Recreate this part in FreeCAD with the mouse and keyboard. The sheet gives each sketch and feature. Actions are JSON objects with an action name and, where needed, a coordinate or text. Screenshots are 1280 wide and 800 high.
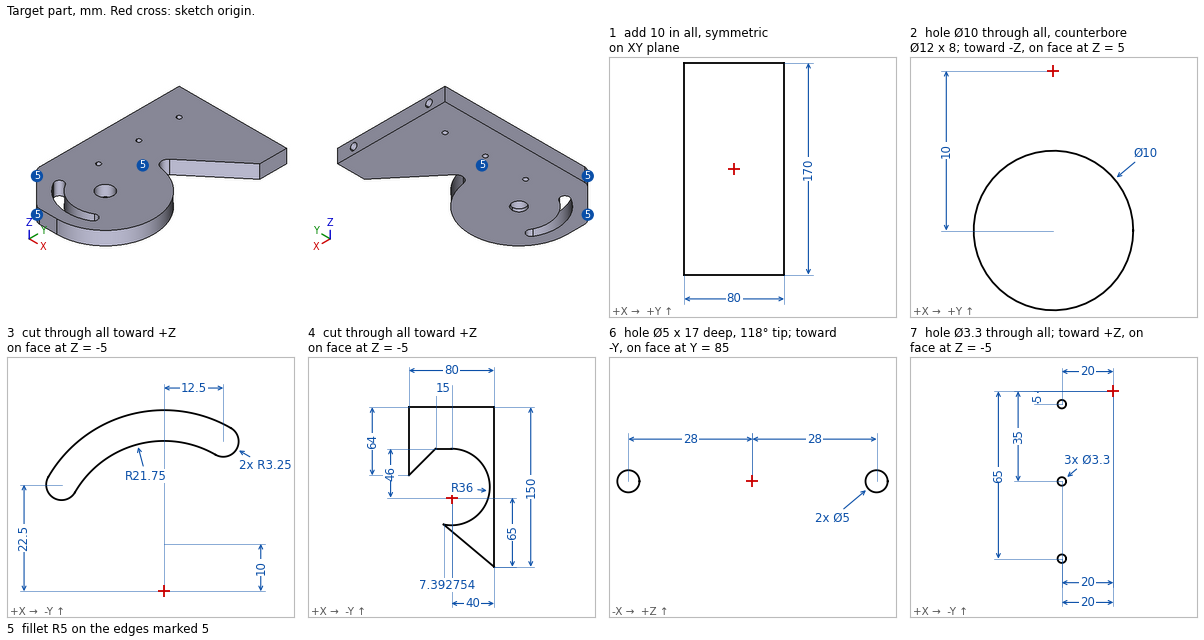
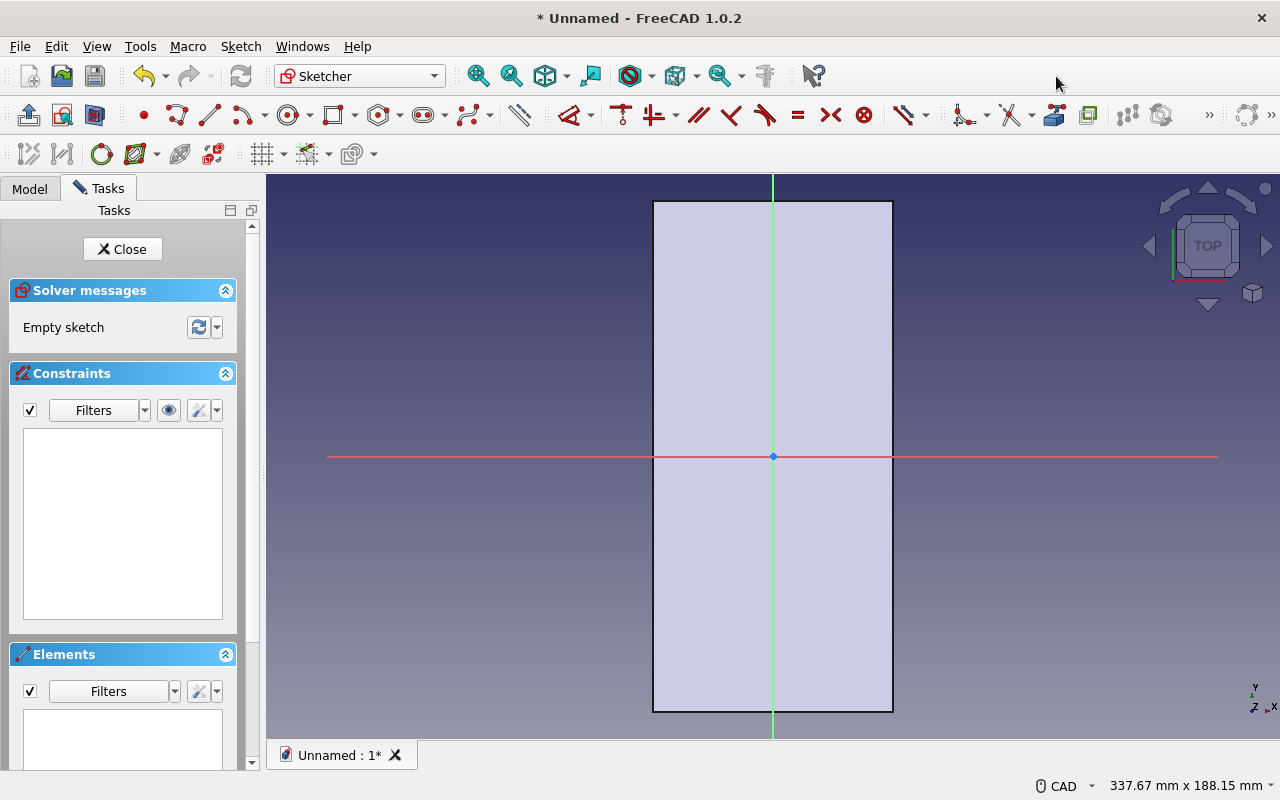
{"action": "scroll", "coordinate": [784, 483], "scroll_direction": "up", "scroll_amount": 10}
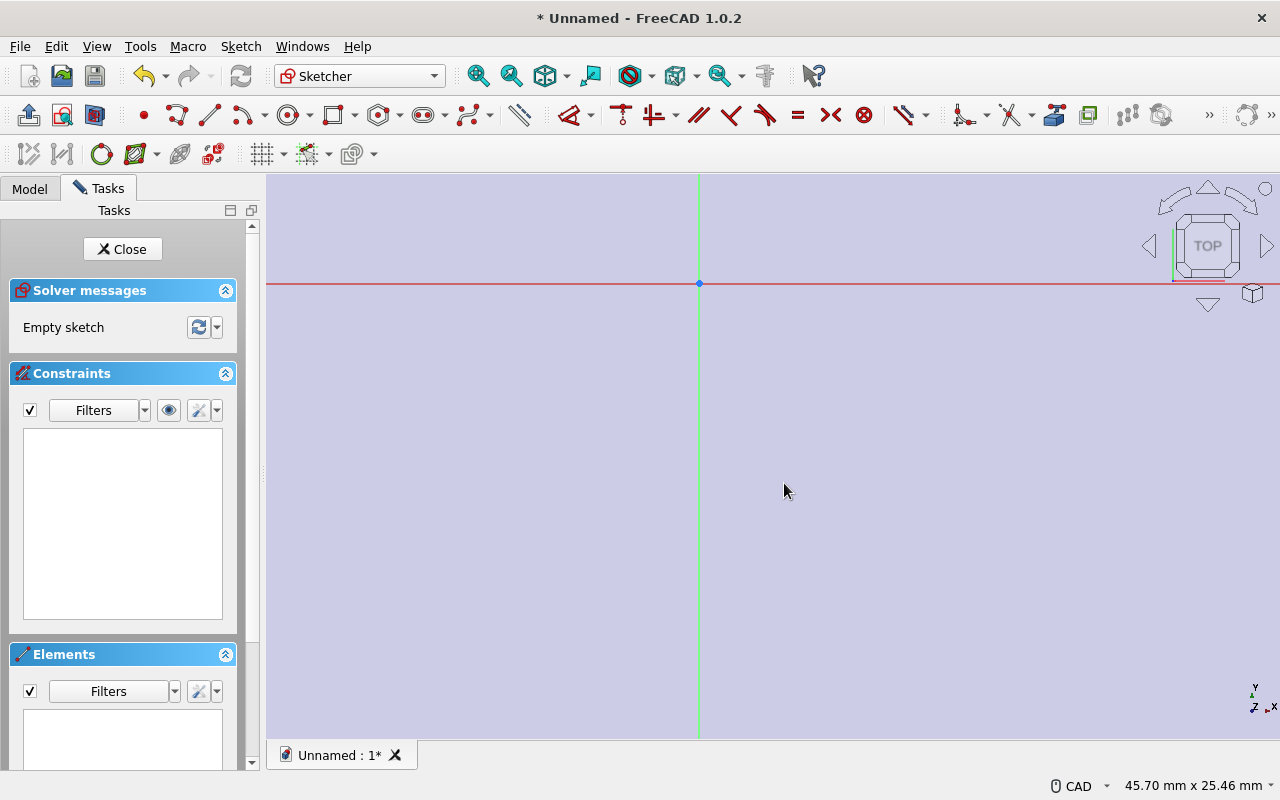
{"action": "left_click", "coordinate": [288, 116]}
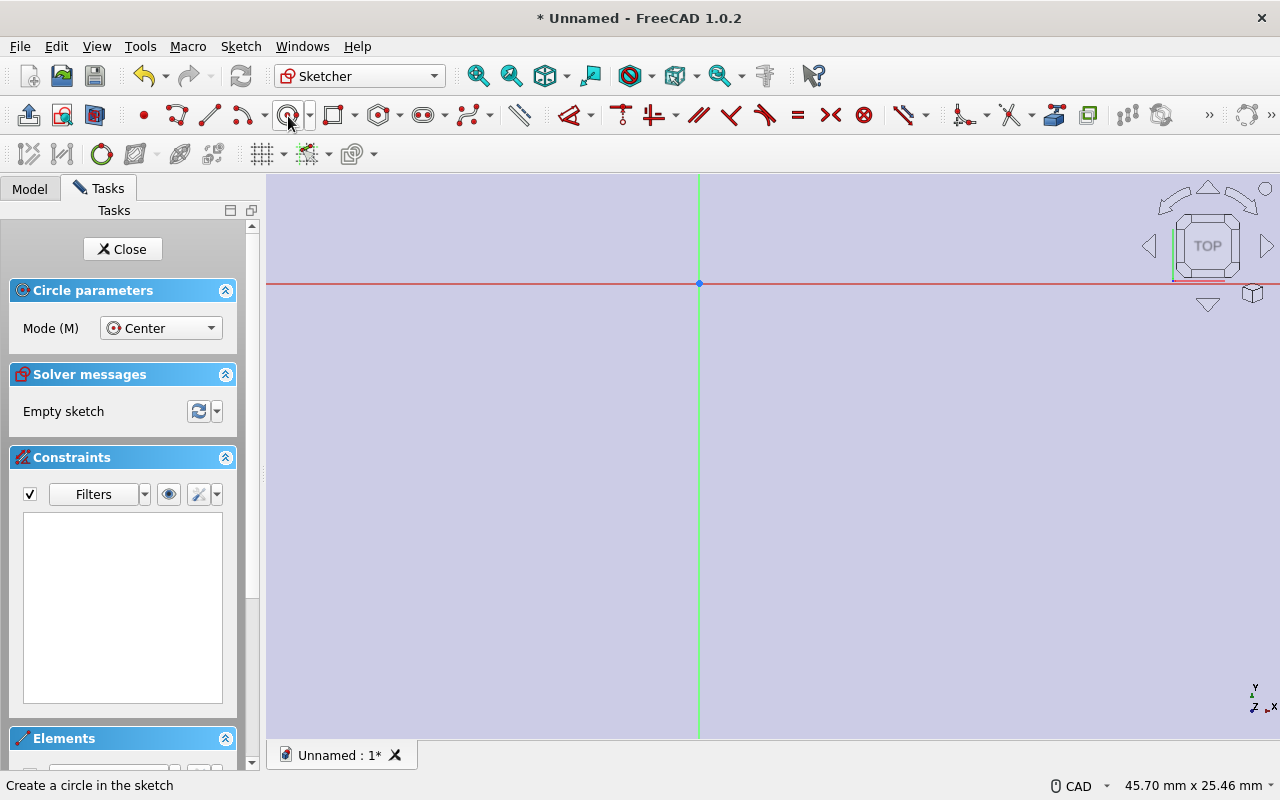
{"action": "left_click", "coordinate": [699, 506]}
{"action": "left_click", "coordinate": [778, 427]}
{"action": "key", "text": "Escape"}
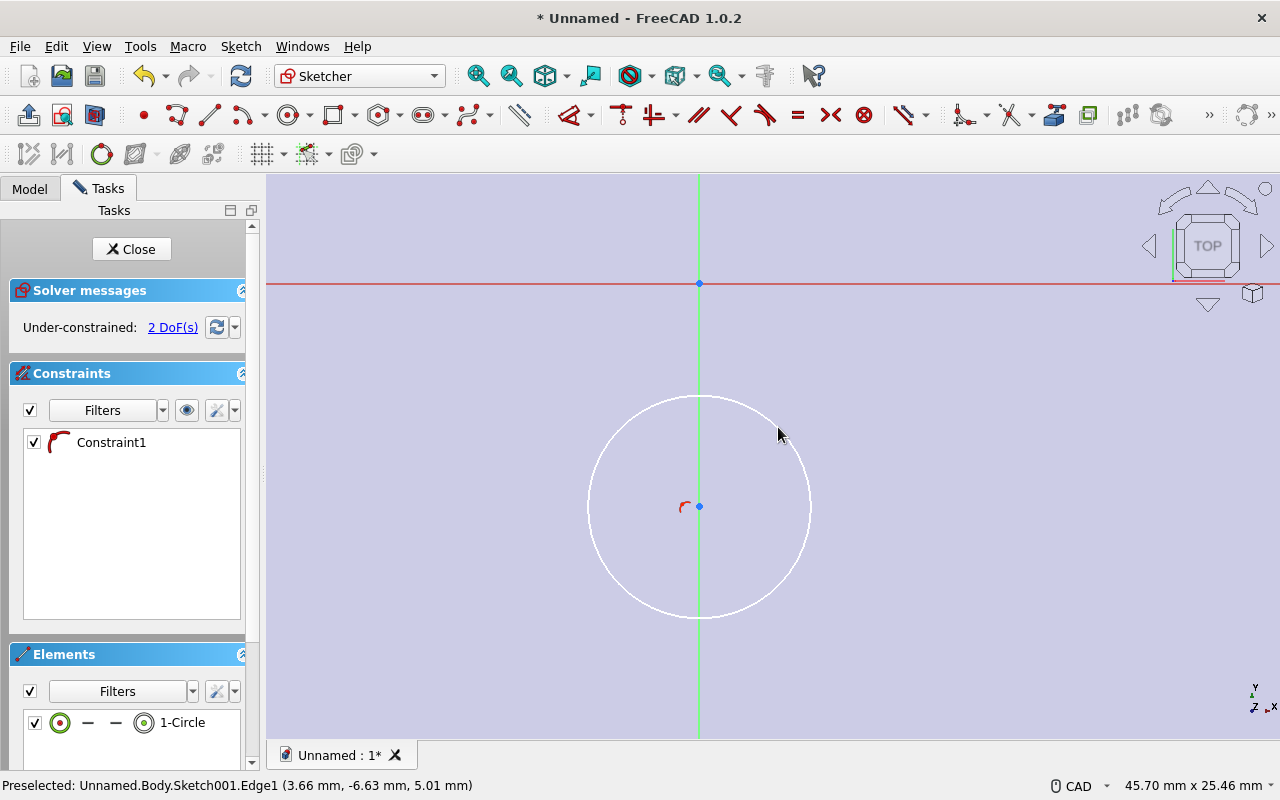
{"action": "key", "text": "d"}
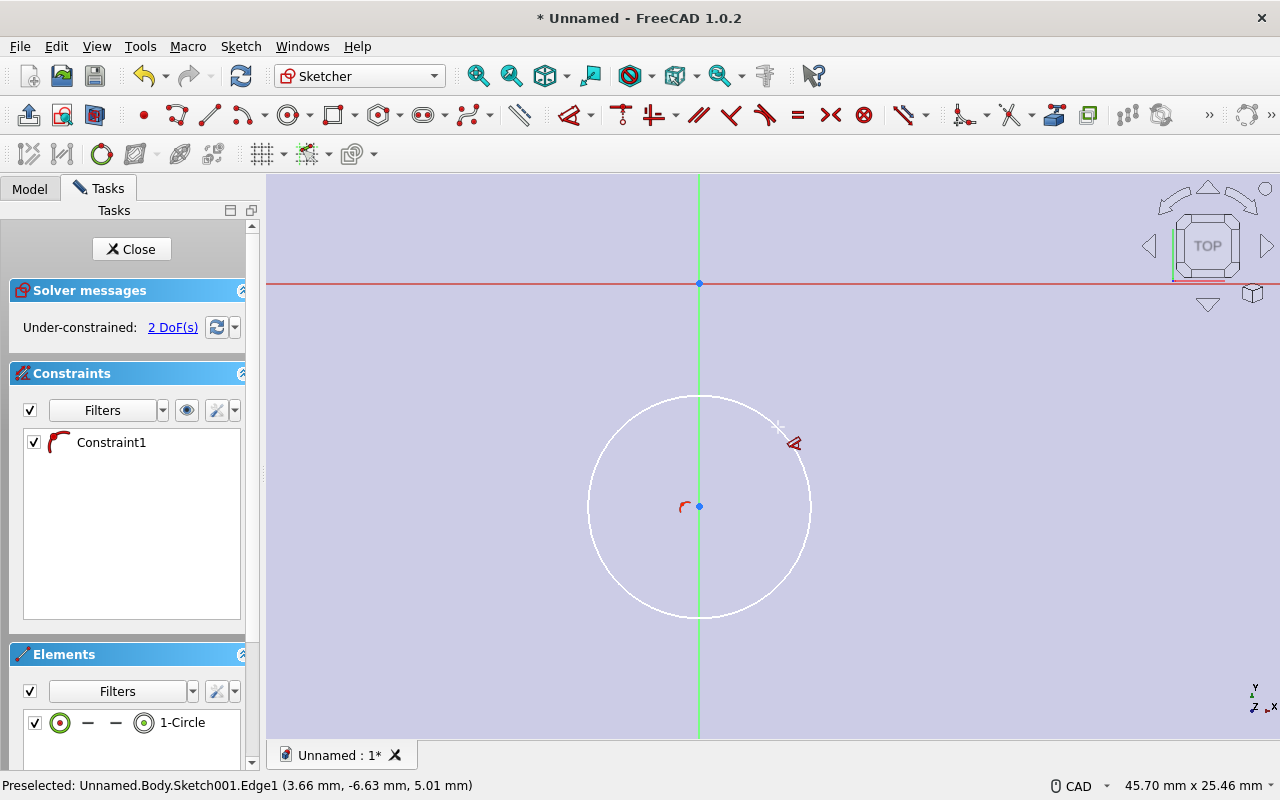
{"action": "left_click", "coordinate": [778, 428]}
{"action": "left_click", "coordinate": [801, 405]}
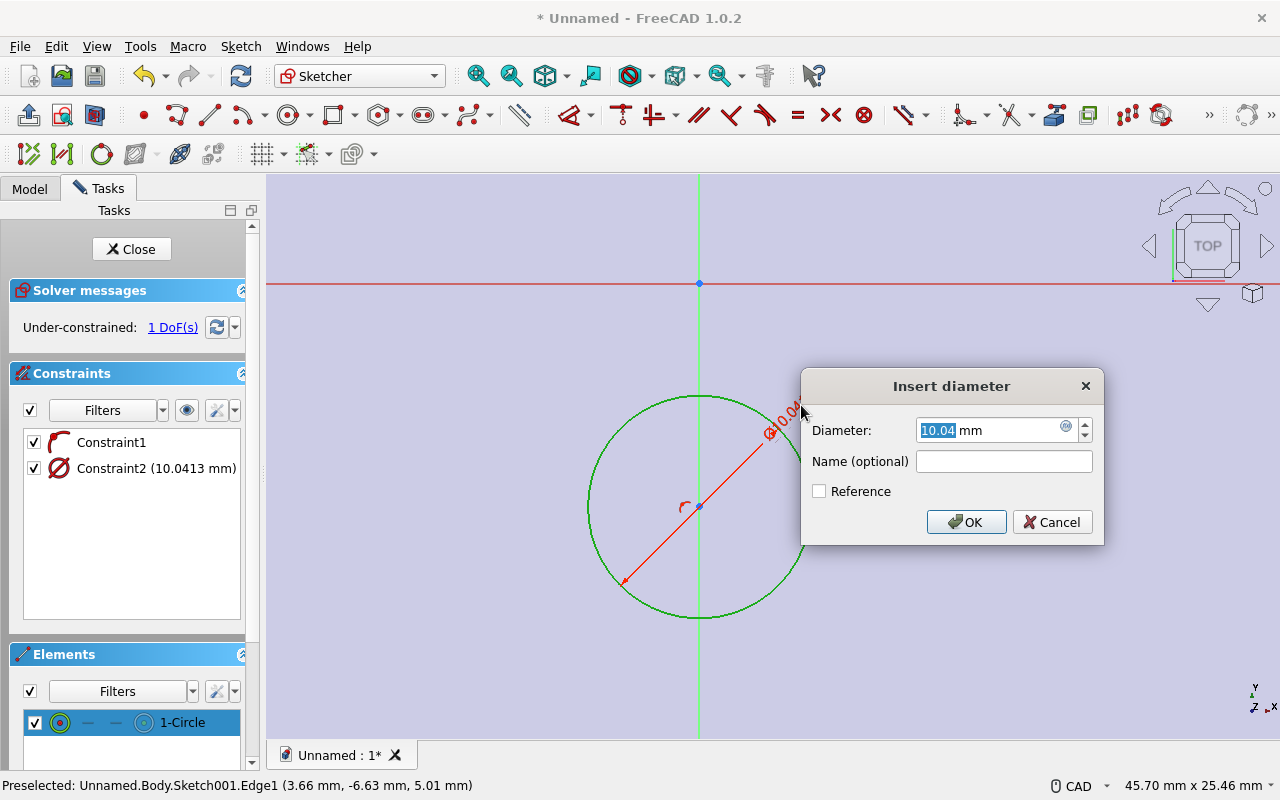
{"action": "type", "text": "10"}
{"action": "key", "text": "Return"}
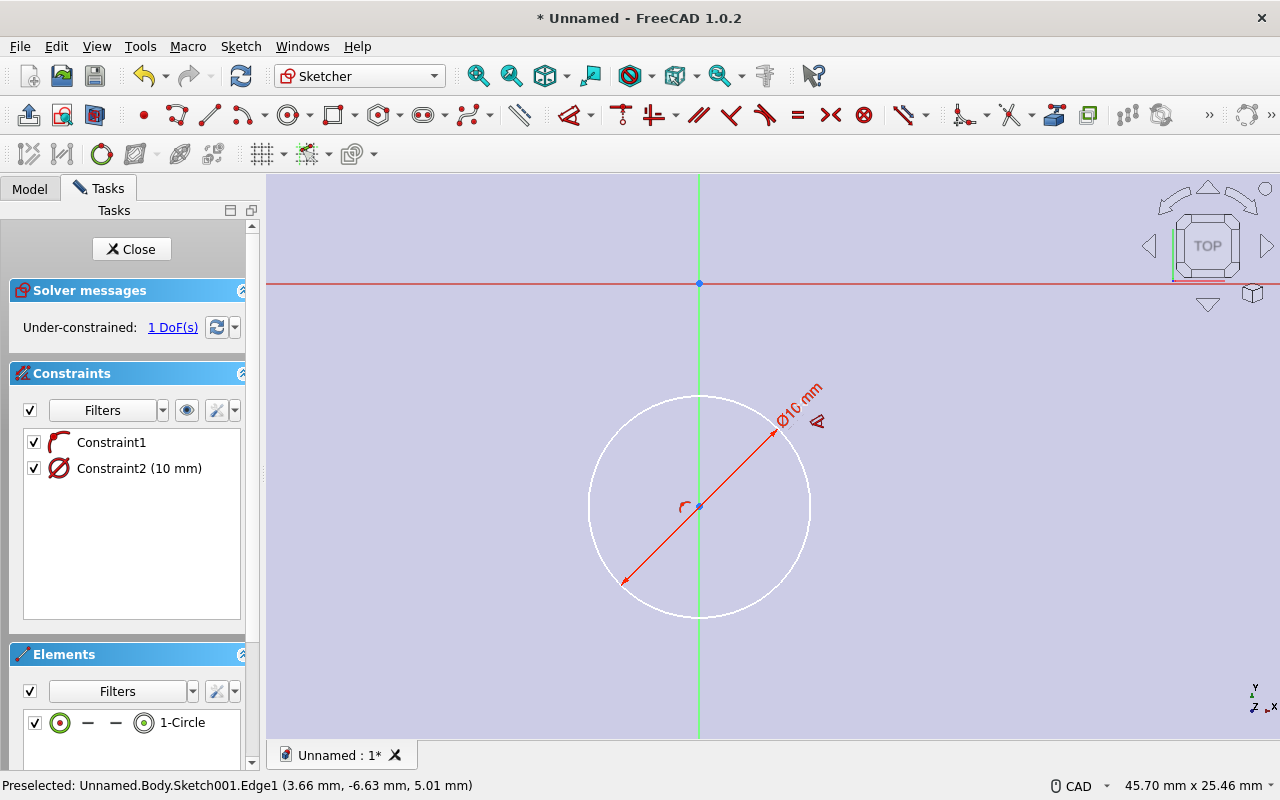
{"action": "left_click", "coordinate": [699, 507]}
{"action": "left_click", "coordinate": [733, 344]}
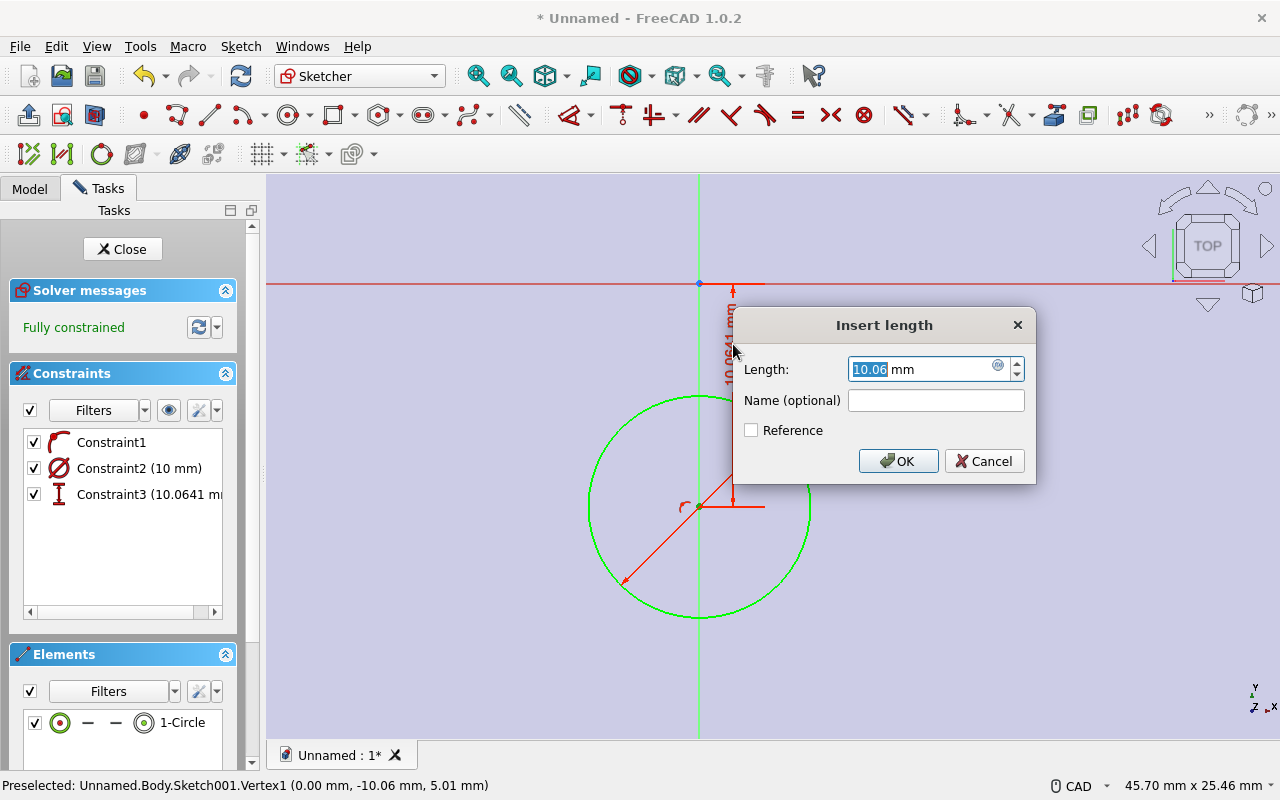
{"action": "type", "text": "10"}
{"action": "key", "text": "Return"}
{"action": "key", "text": "Escape"}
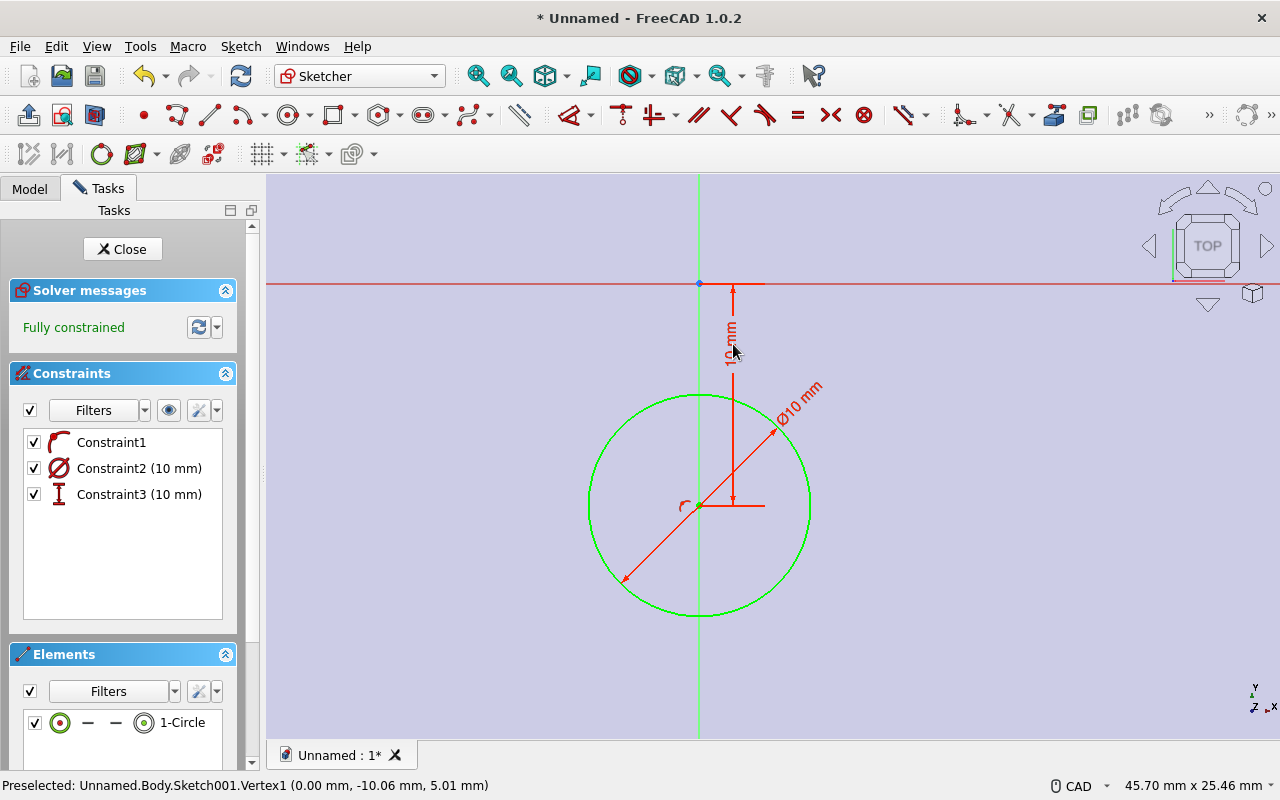
{"action": "left_click", "coordinate": [123, 249]}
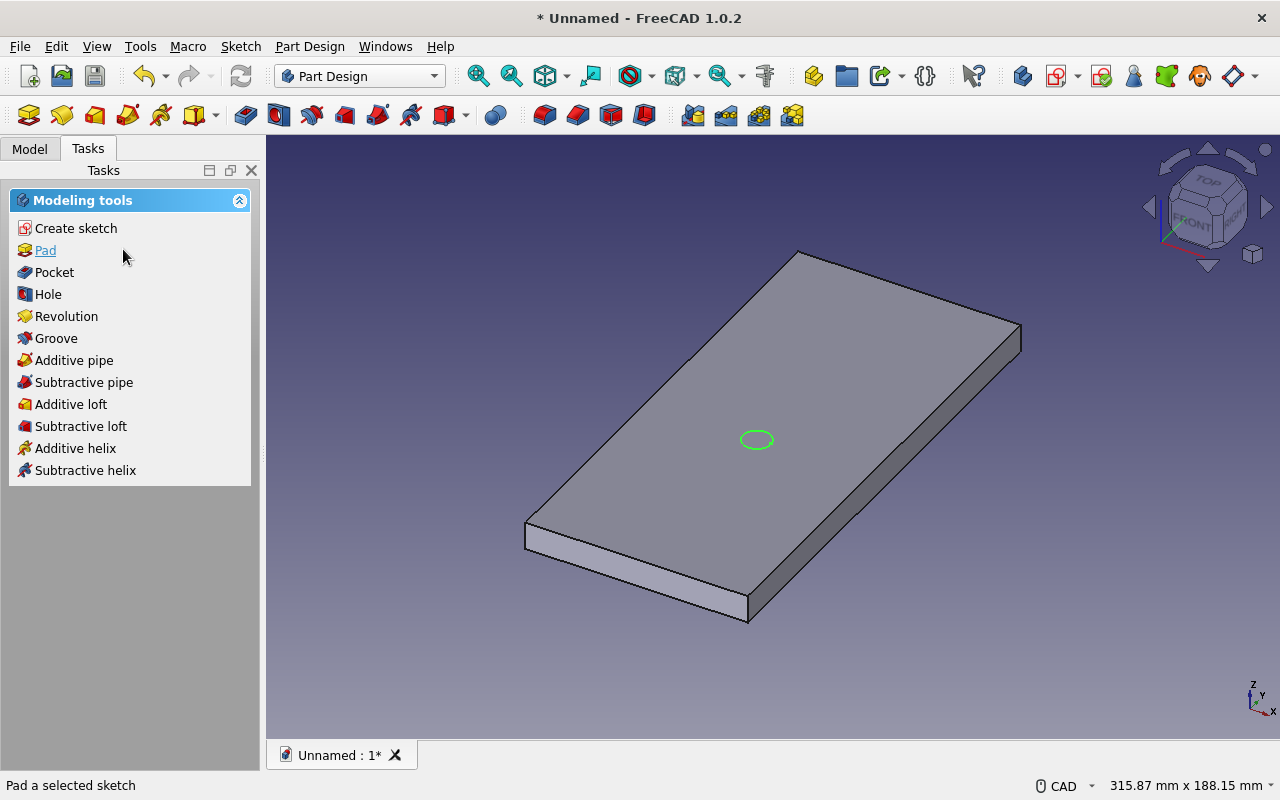
{"action": "left_click", "coordinate": [279, 116]}